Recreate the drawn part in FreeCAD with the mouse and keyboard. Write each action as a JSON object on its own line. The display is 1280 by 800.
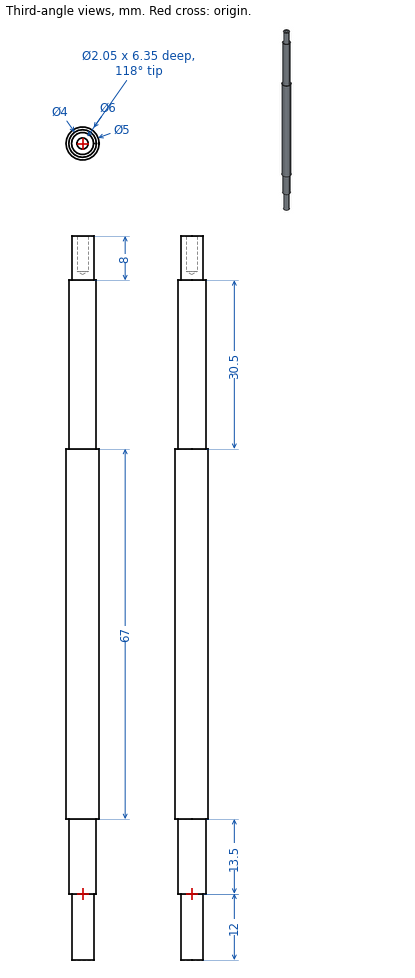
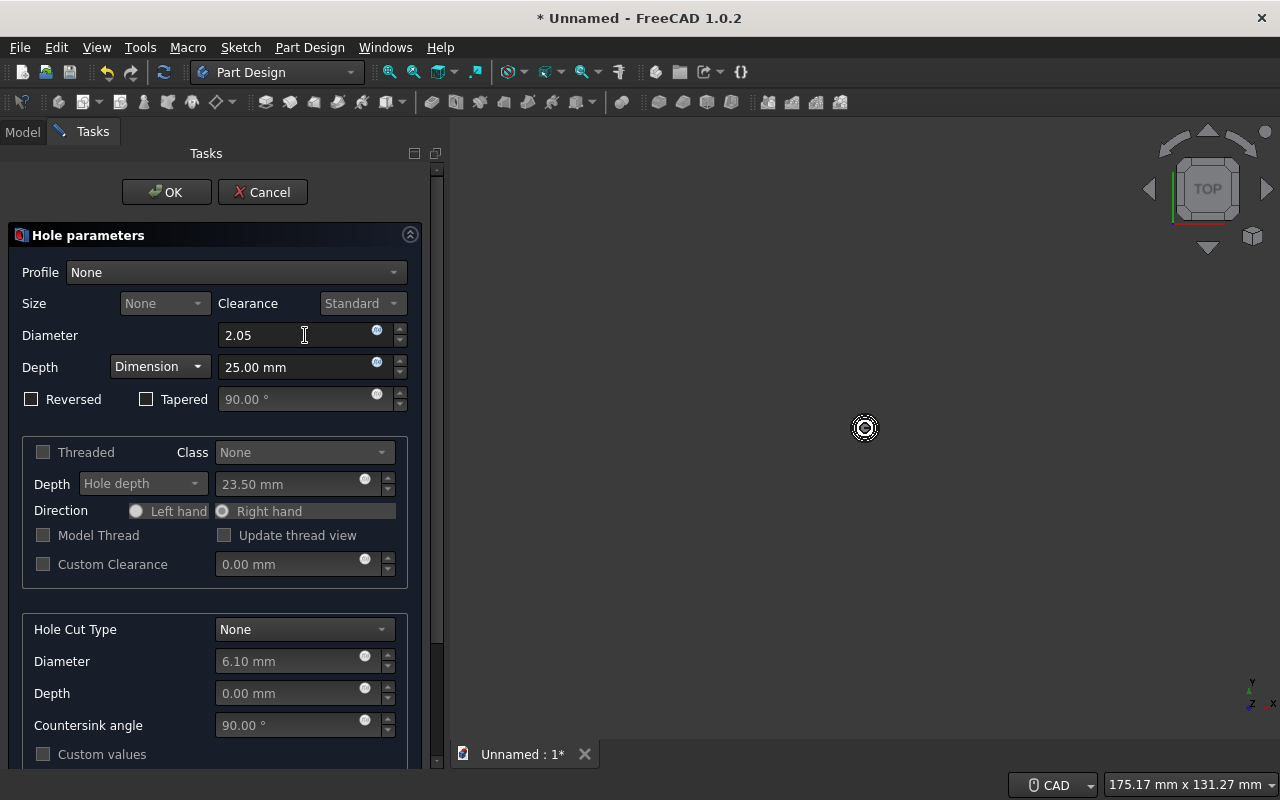
{"action": "triple_click", "coordinate": [305, 367]}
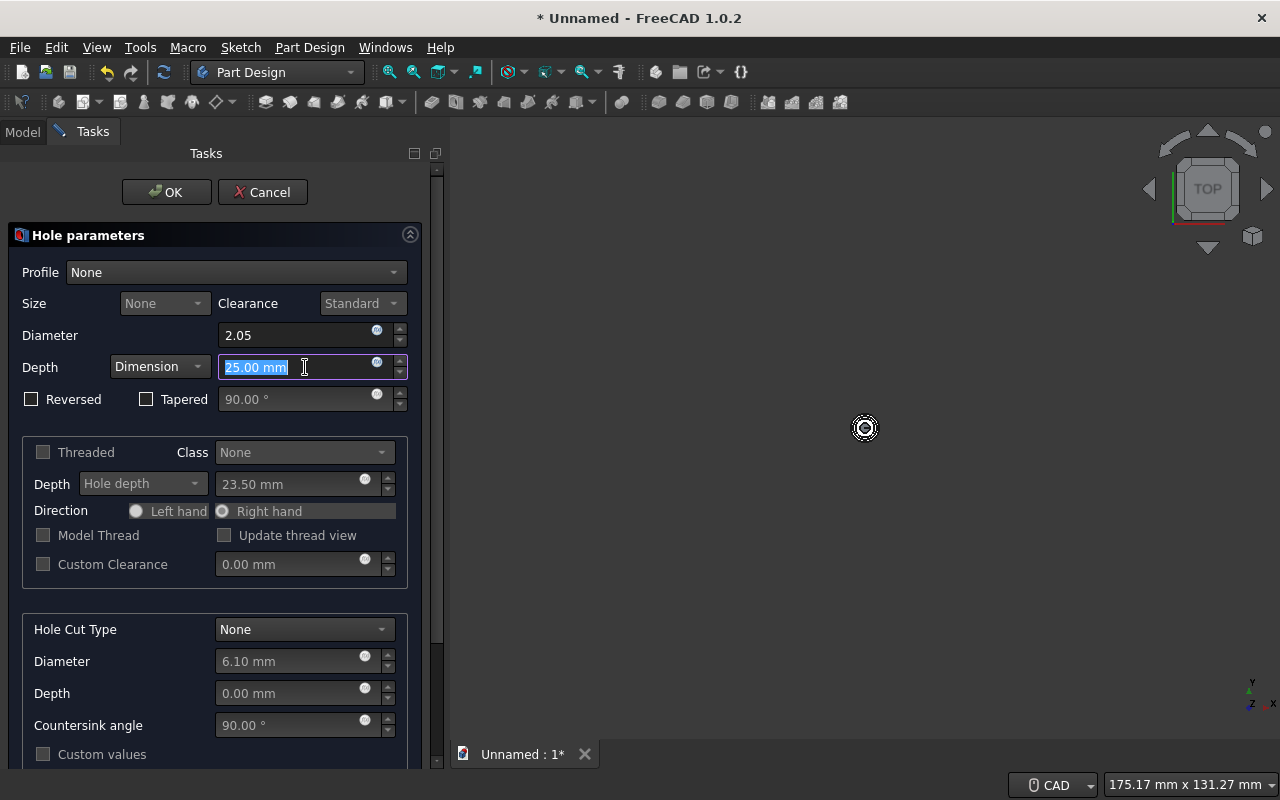
{"action": "type", "text": "6.35"}
{"action": "key", "text": "Tab"}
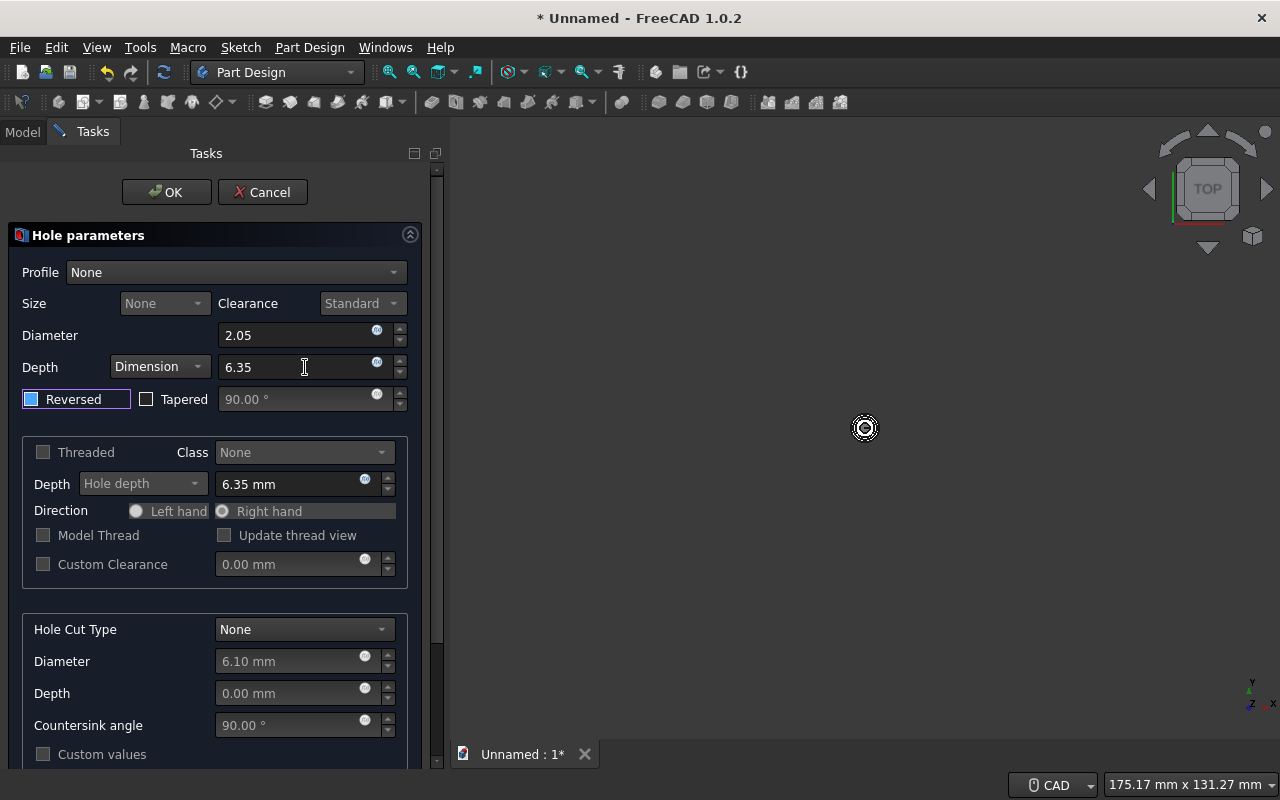
{"action": "left_click", "coordinate": [167, 192]}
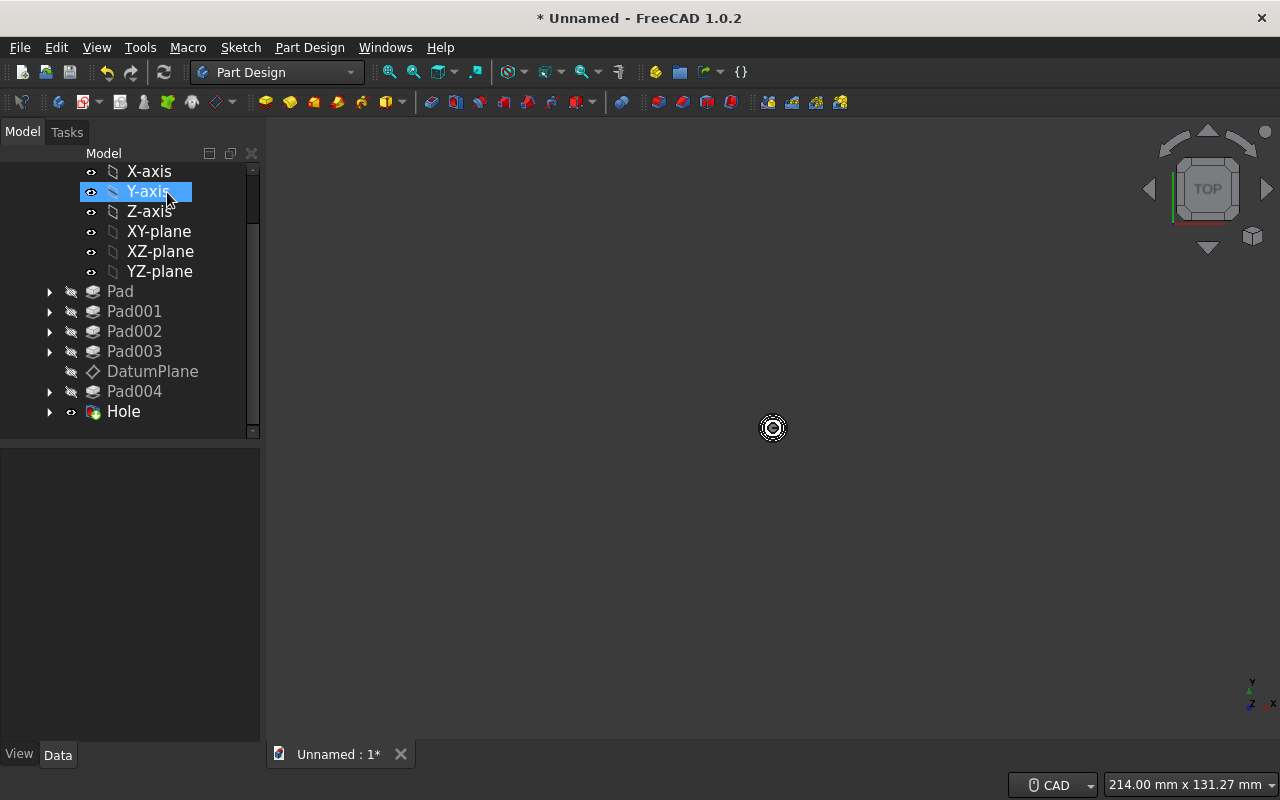
{"action": "key", "text": "0"}